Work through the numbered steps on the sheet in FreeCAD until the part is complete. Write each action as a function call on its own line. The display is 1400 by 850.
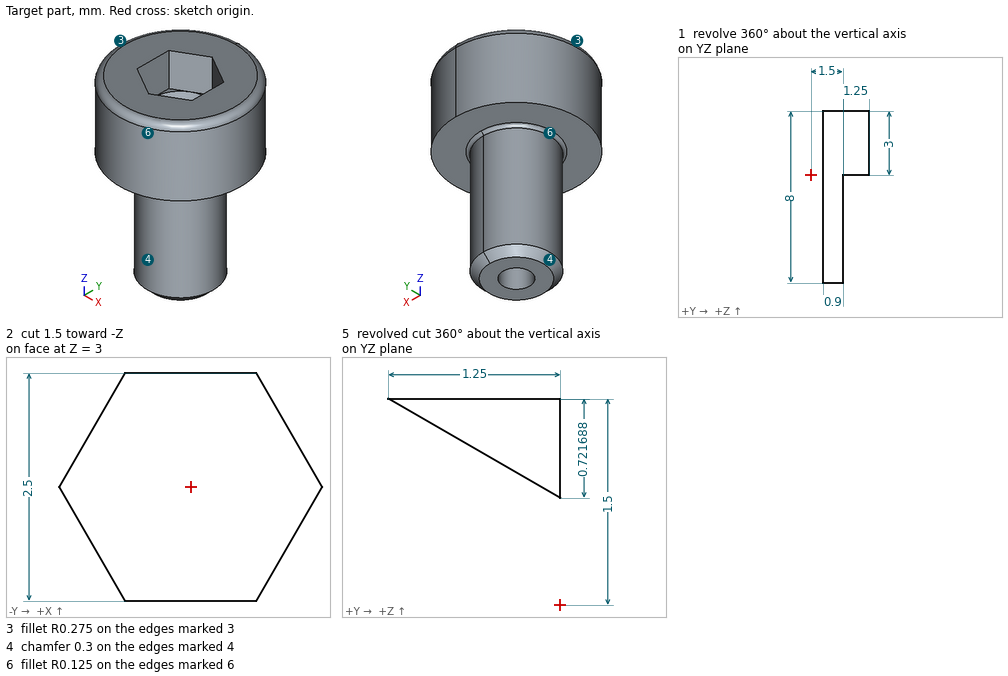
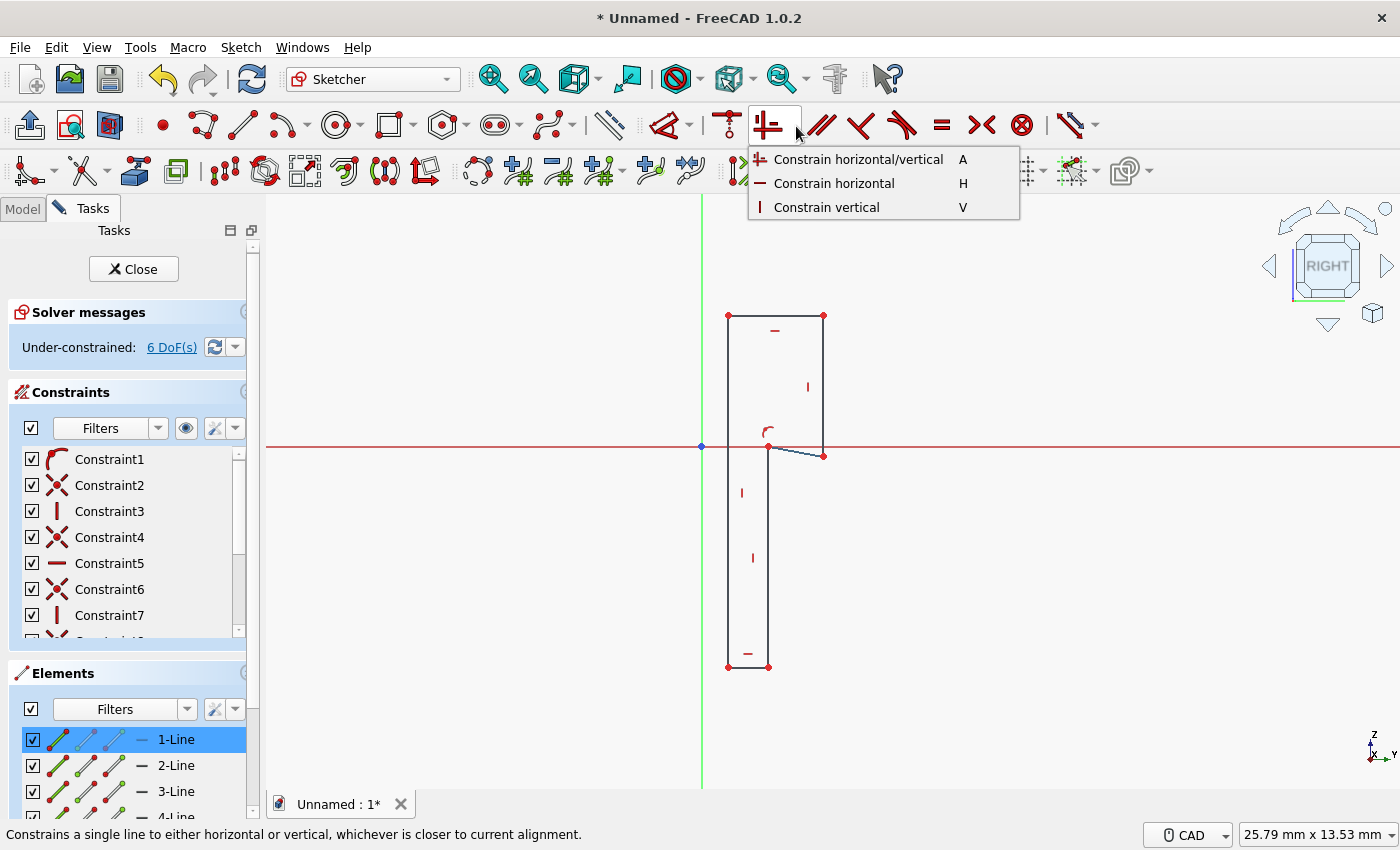
click(884, 183)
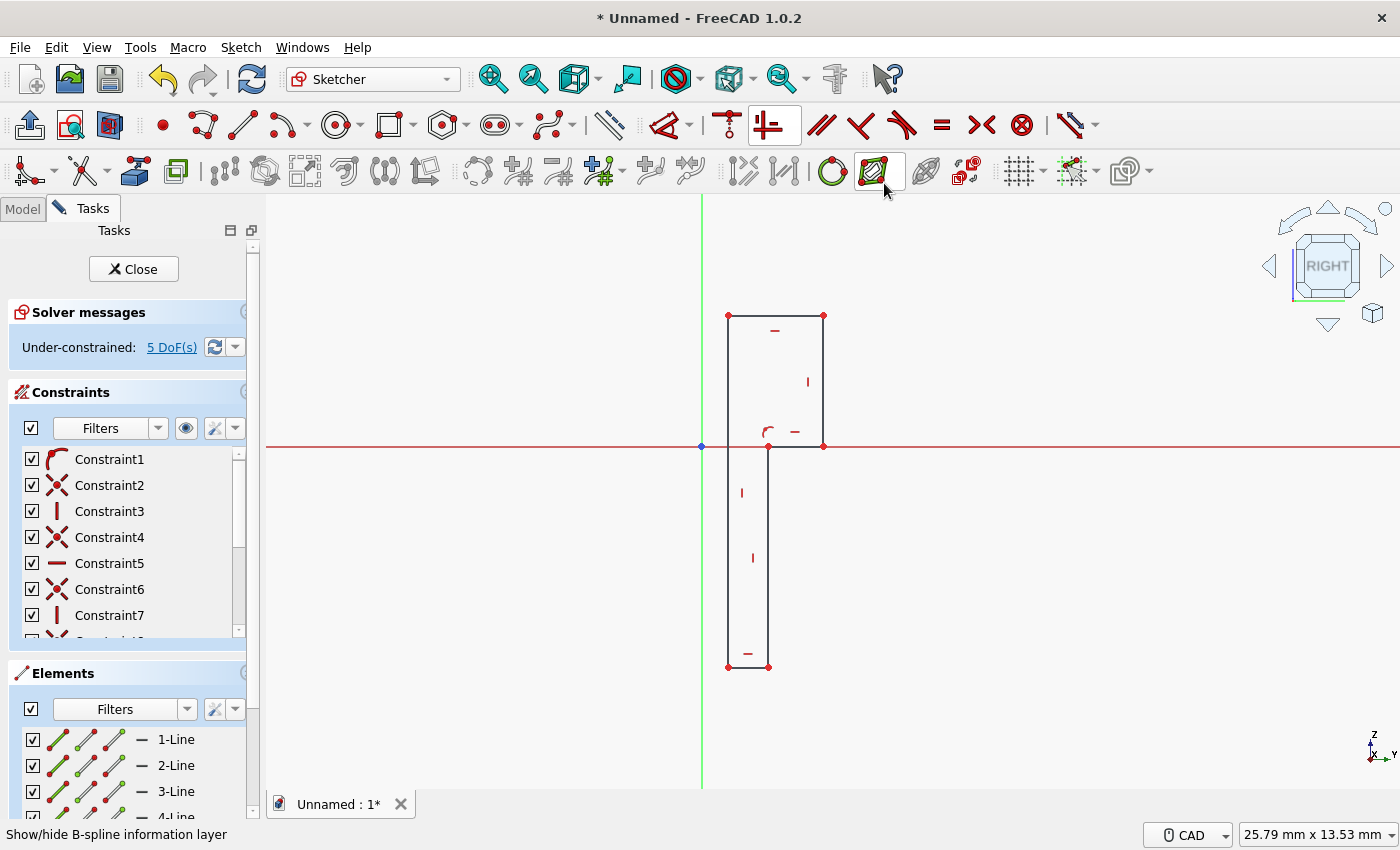
click(664, 126)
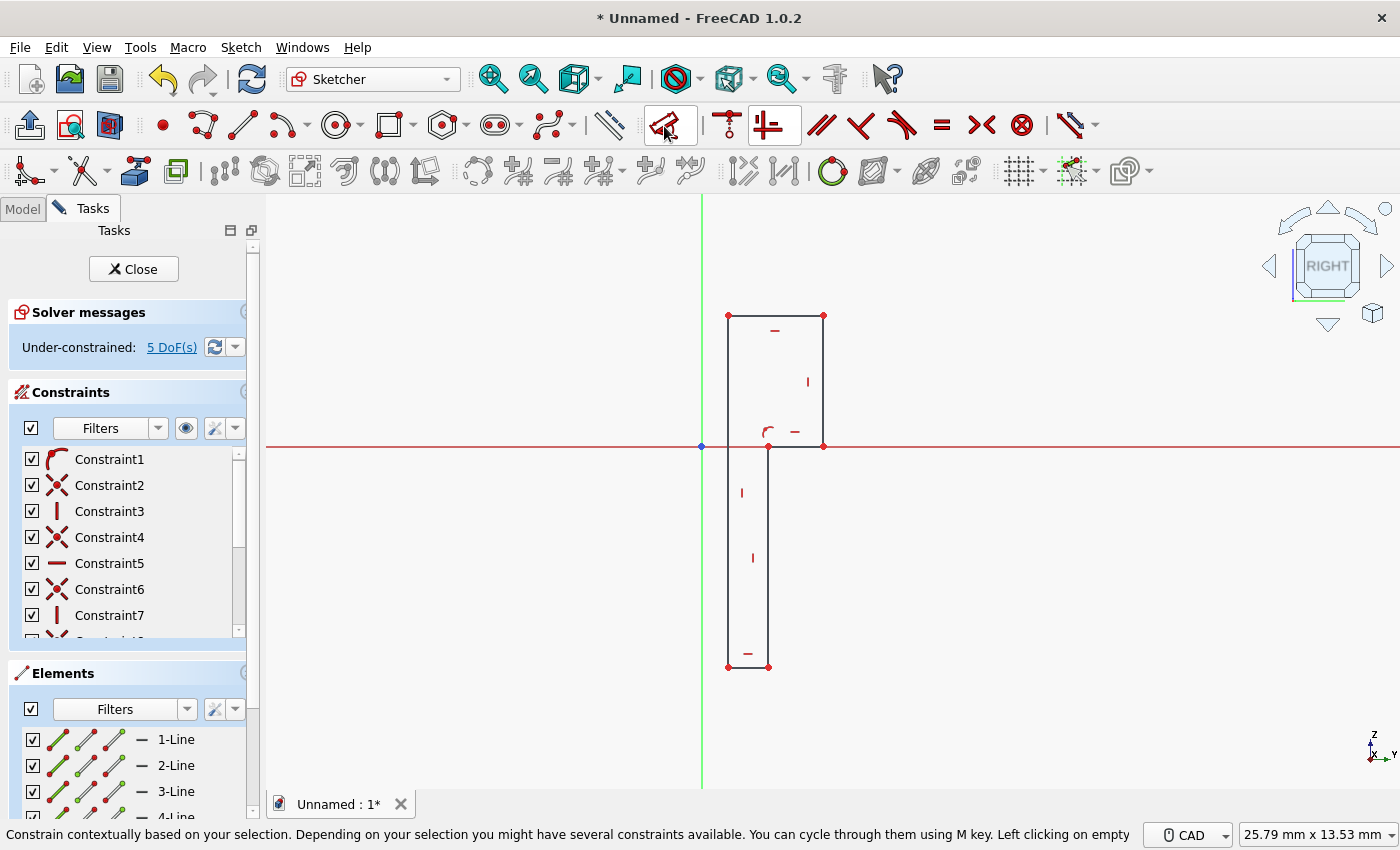
click(823, 407)
click(857, 381)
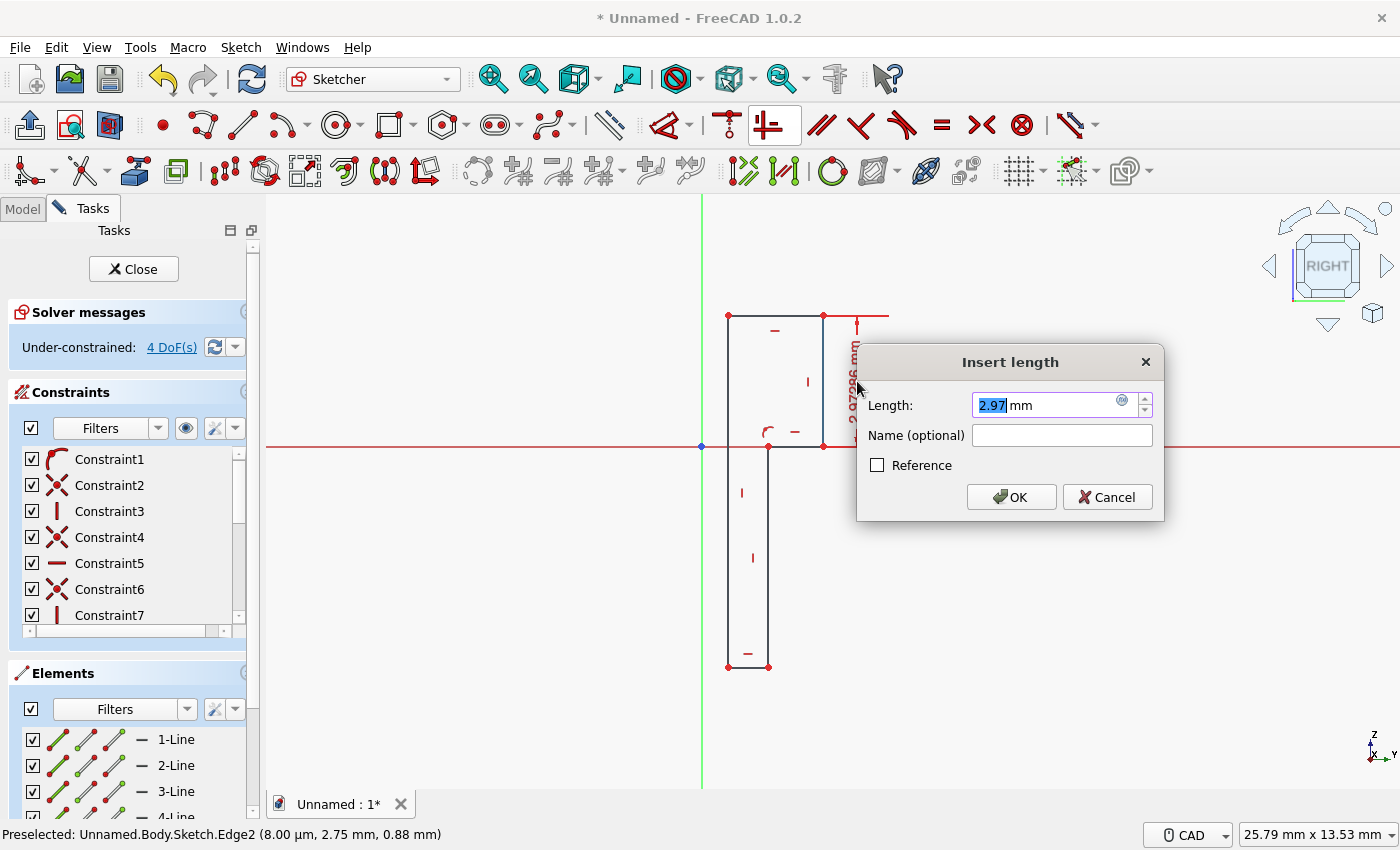
text(3)
key(Return)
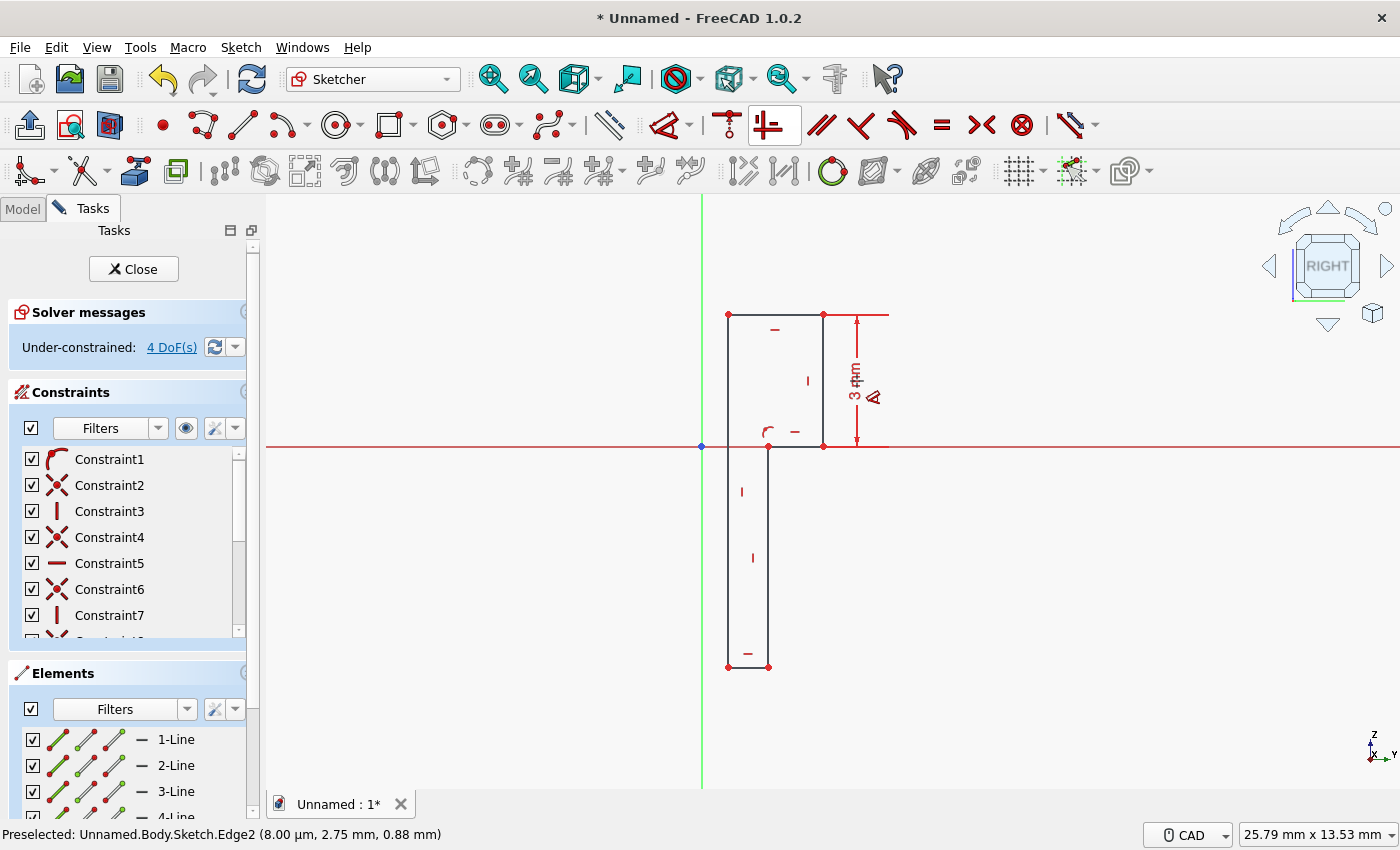
click(728, 421)
click(762, 410)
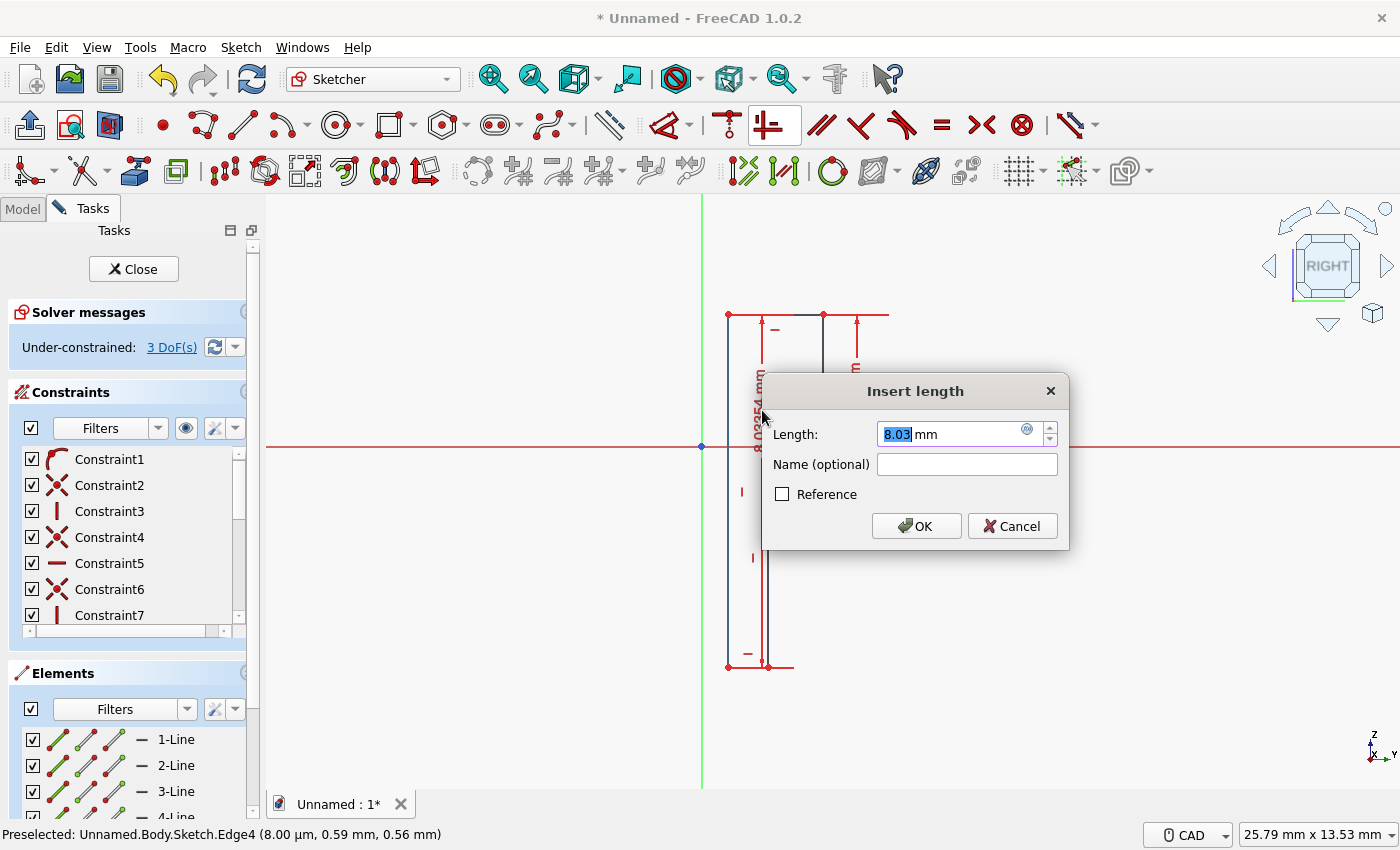
text(8)
key(Return)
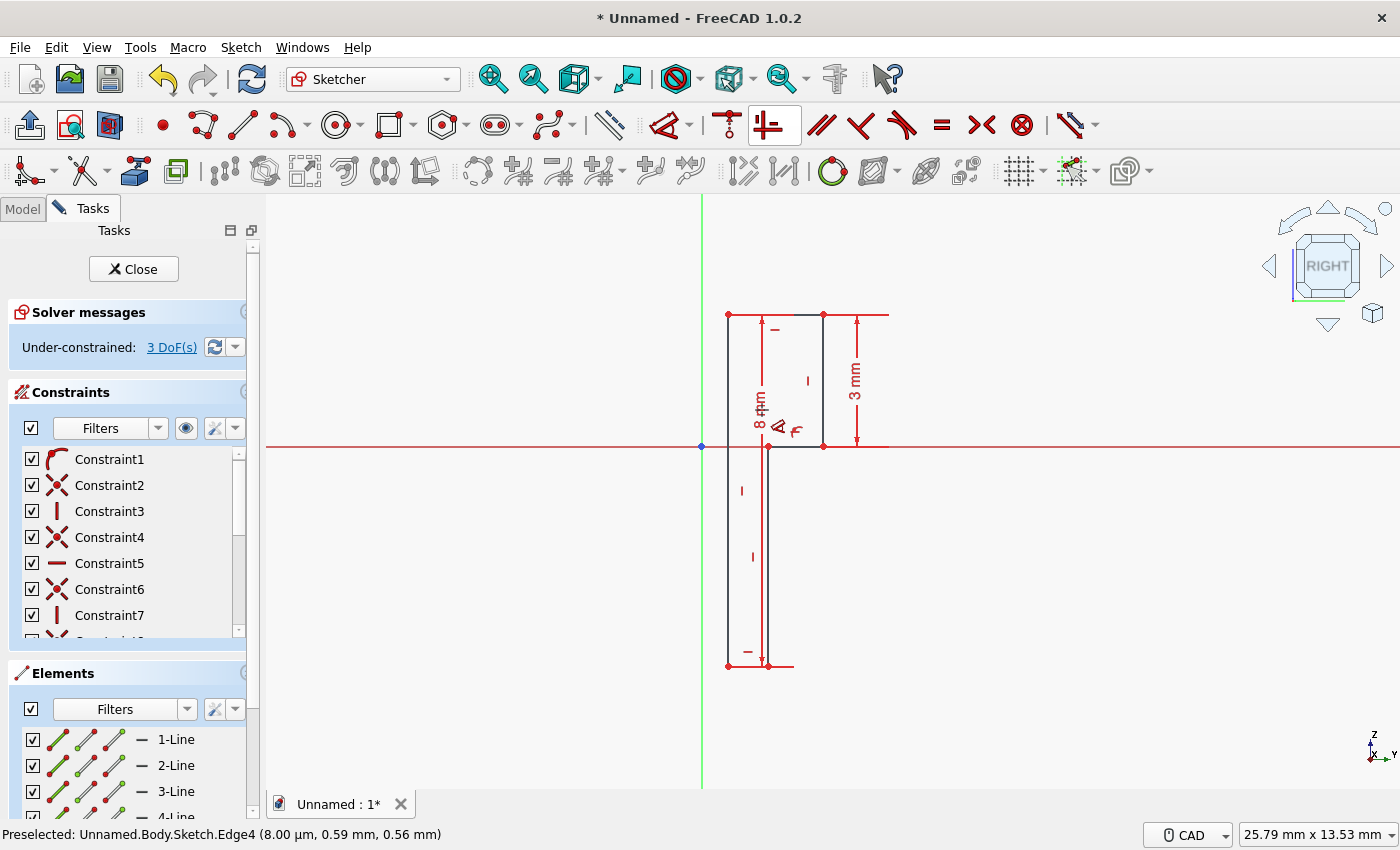
click(740, 667)
click(748, 701)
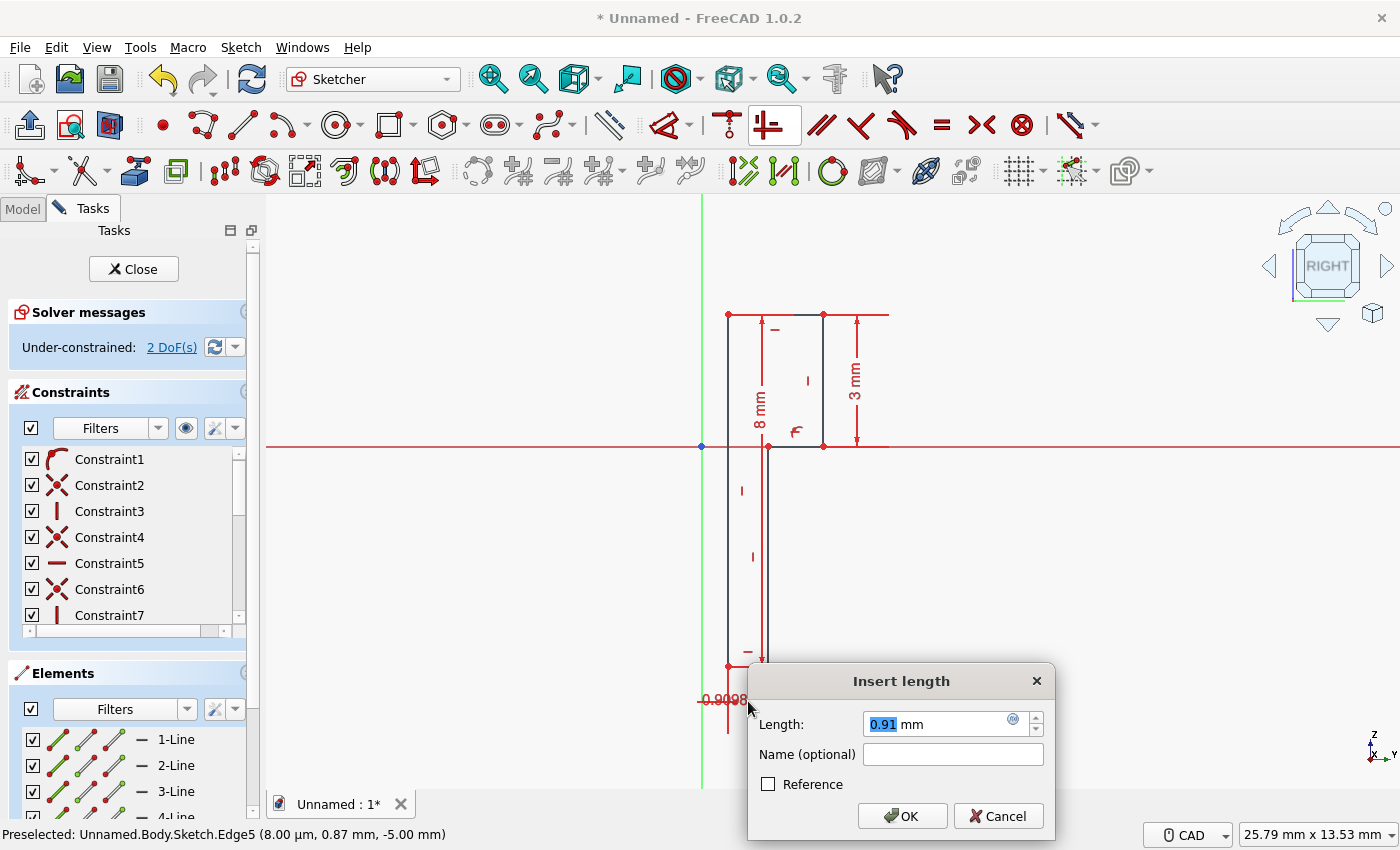
text(0.9)
key(Return)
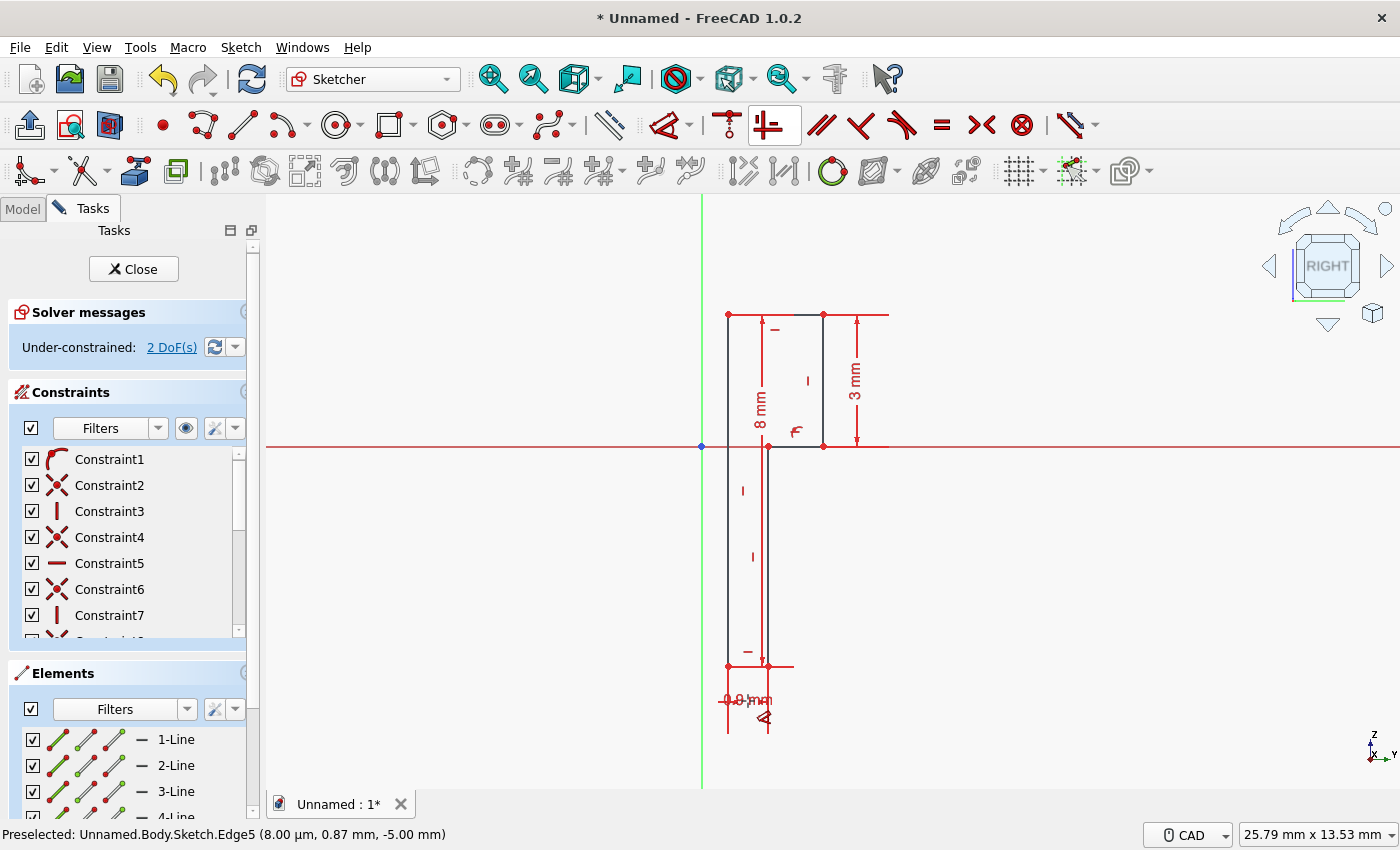
click(785, 447)
click(796, 481)